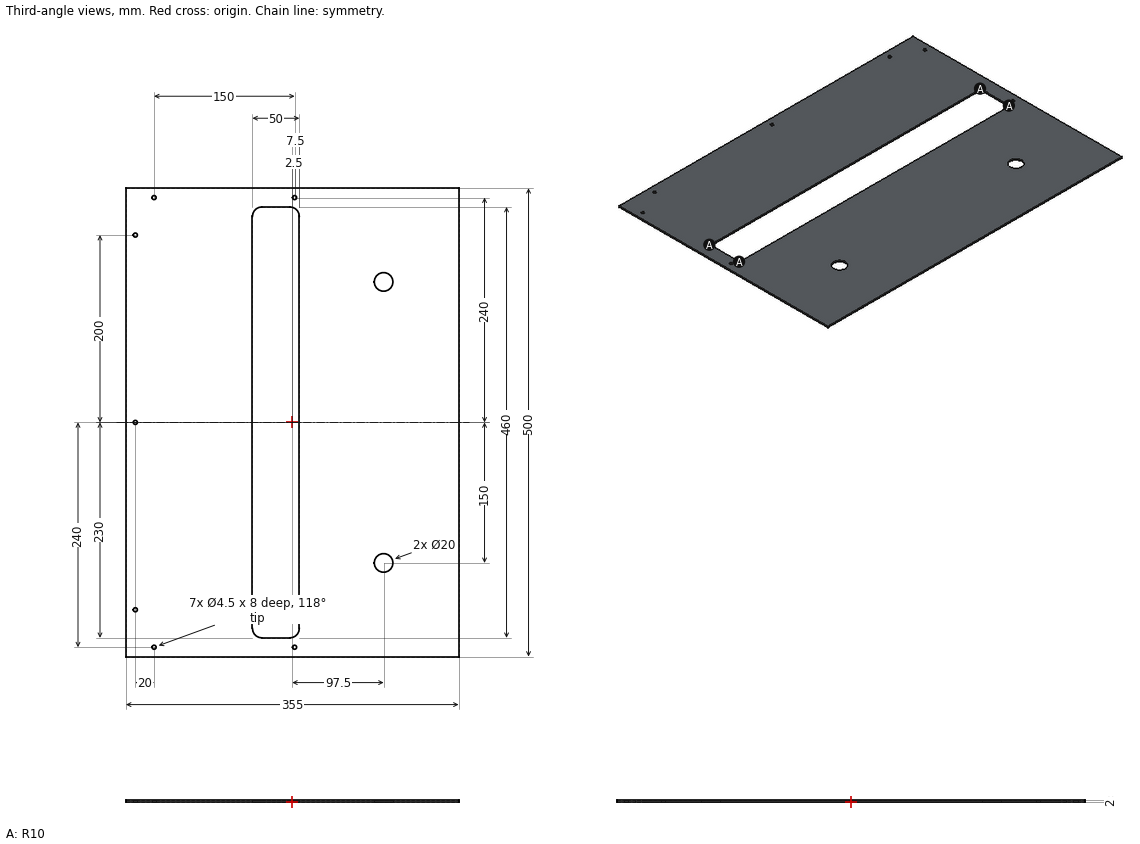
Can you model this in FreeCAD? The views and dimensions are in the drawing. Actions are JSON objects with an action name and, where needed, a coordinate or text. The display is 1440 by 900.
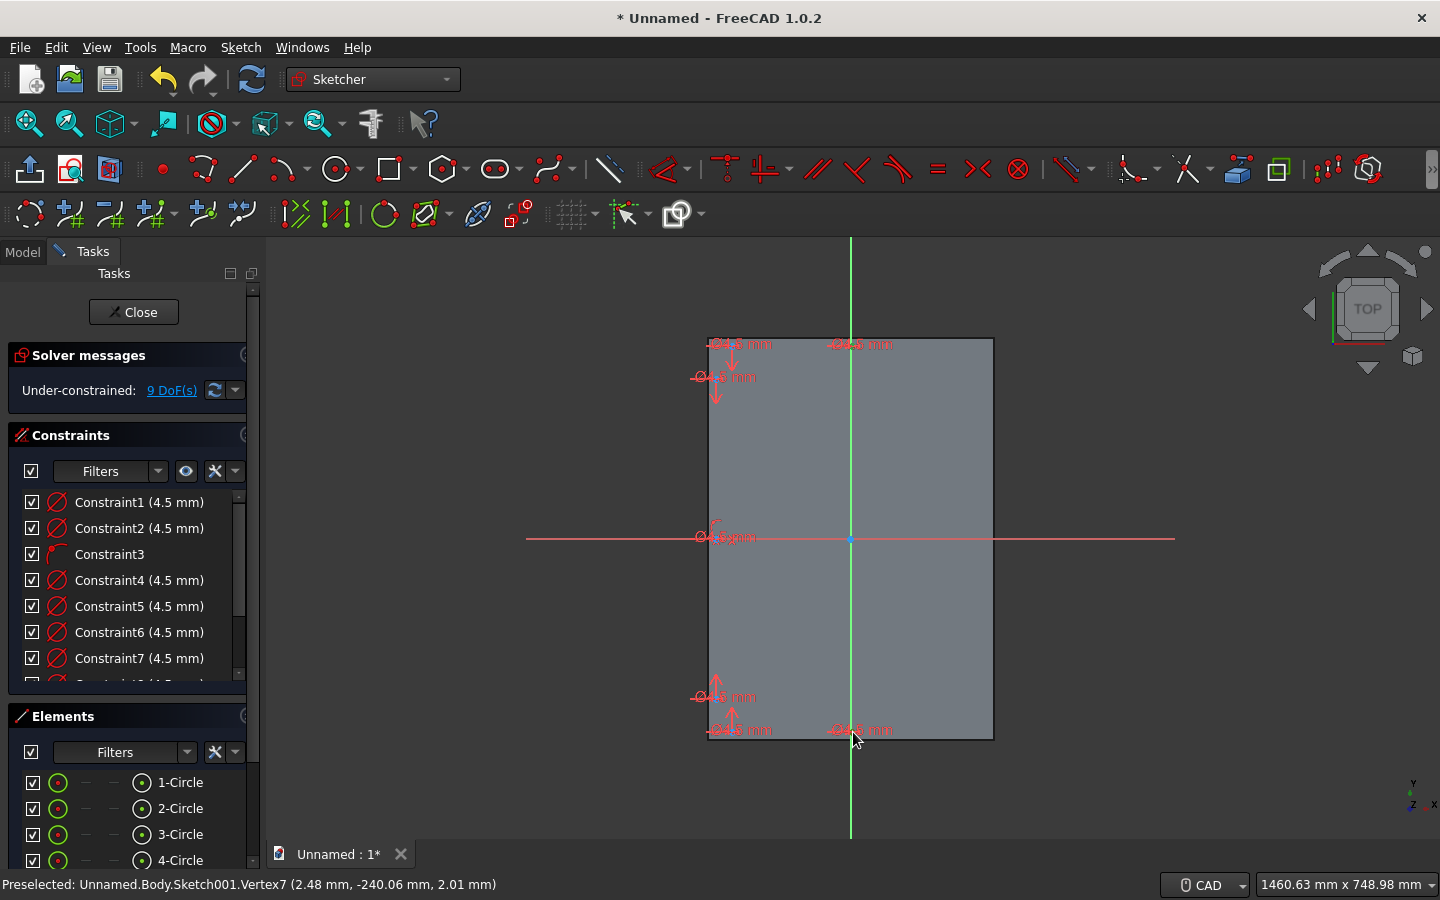
{"action": "left_click", "coordinate": [574, 539]}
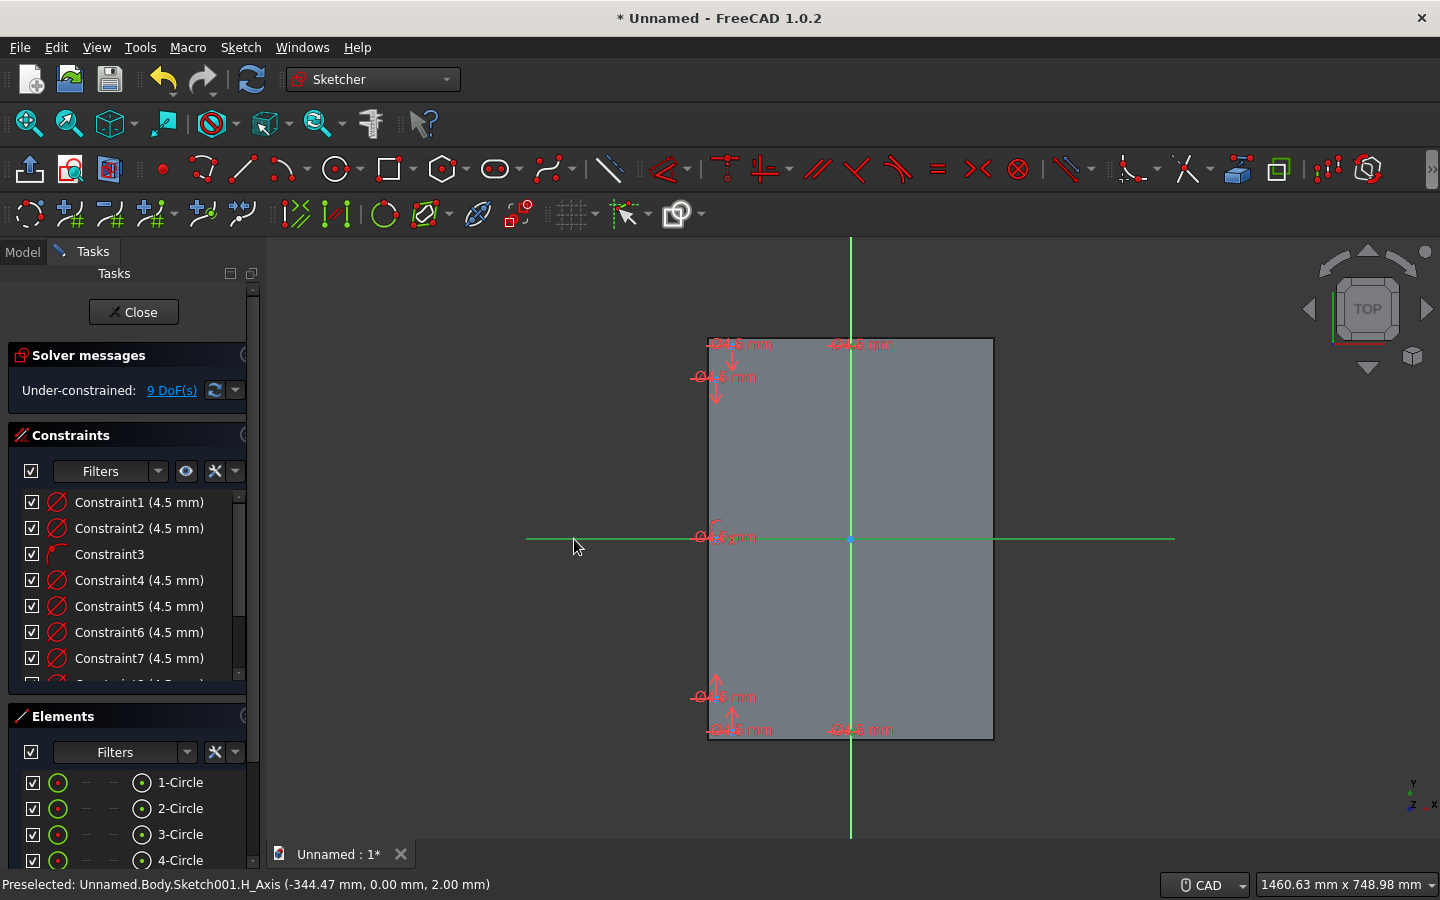
{"action": "key", "text": "s"}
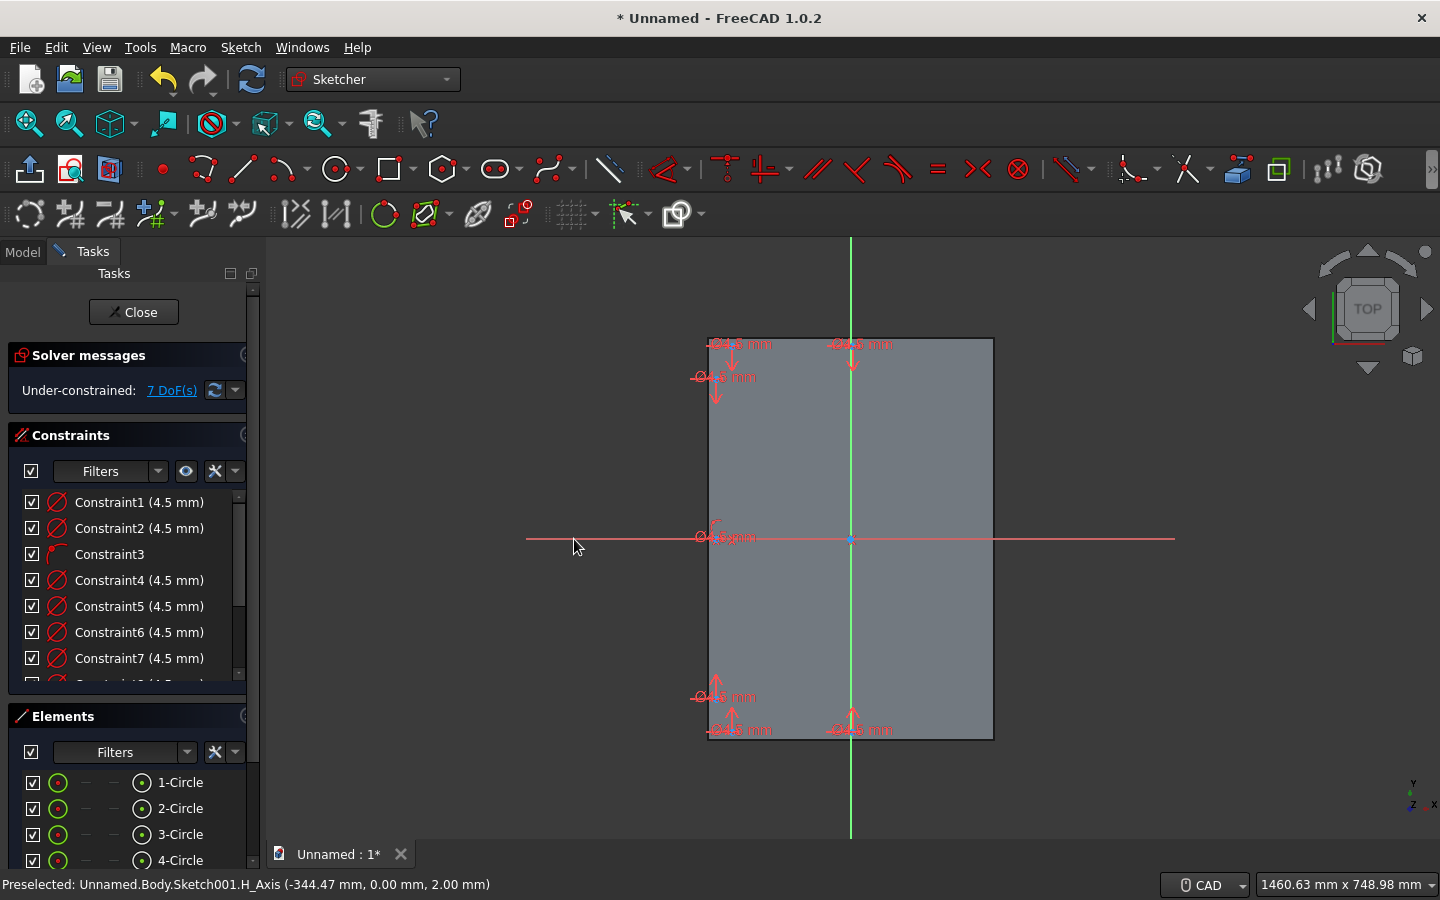
{"action": "left_click", "coordinate": [664, 170]}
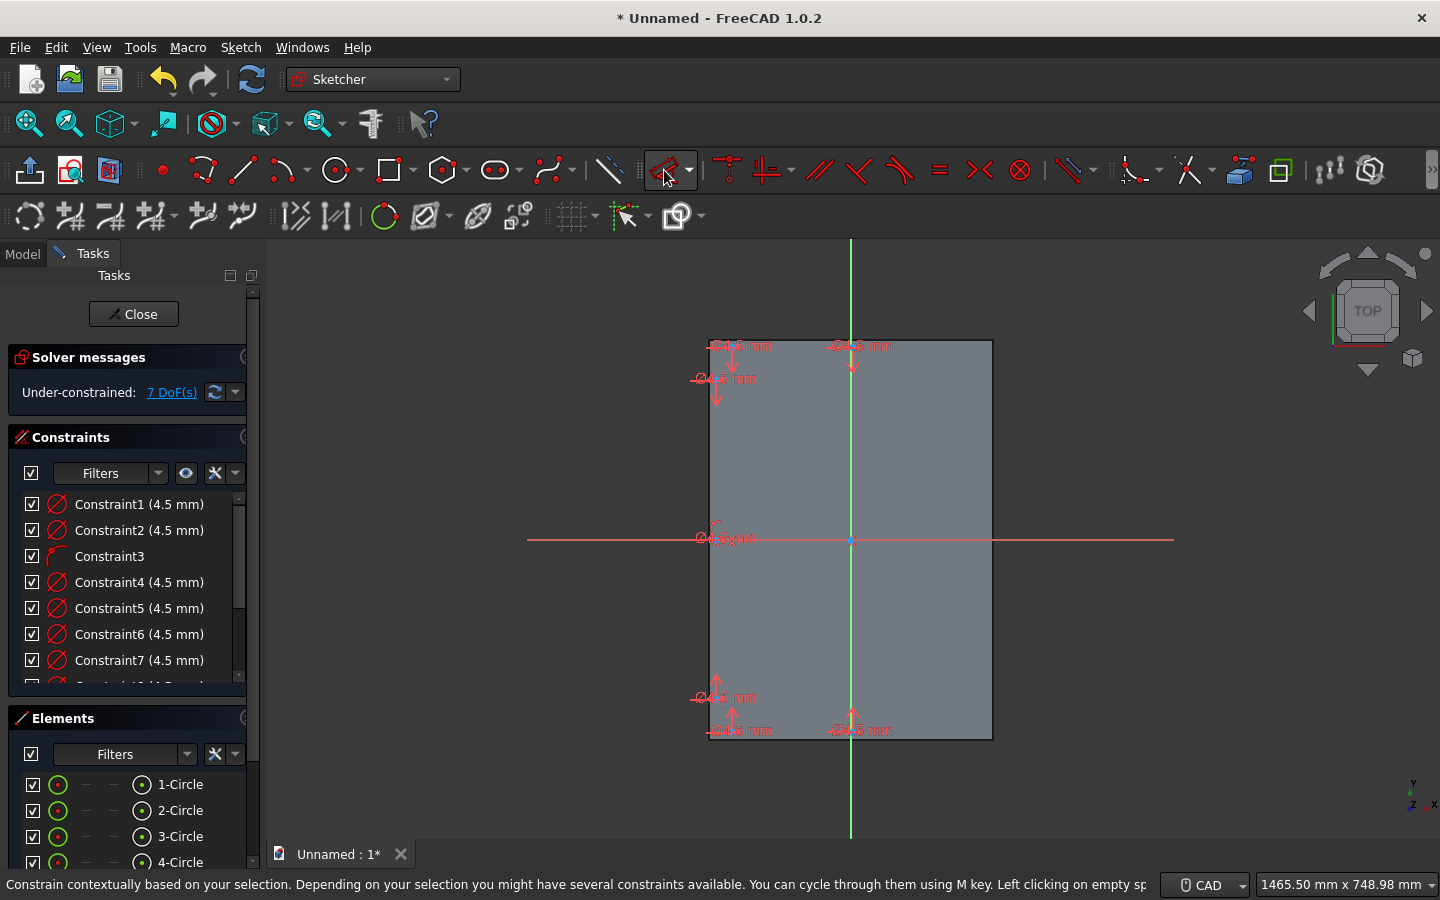
{"action": "left_click", "coordinate": [732, 733]}
{"action": "left_click", "coordinate": [885, 636]}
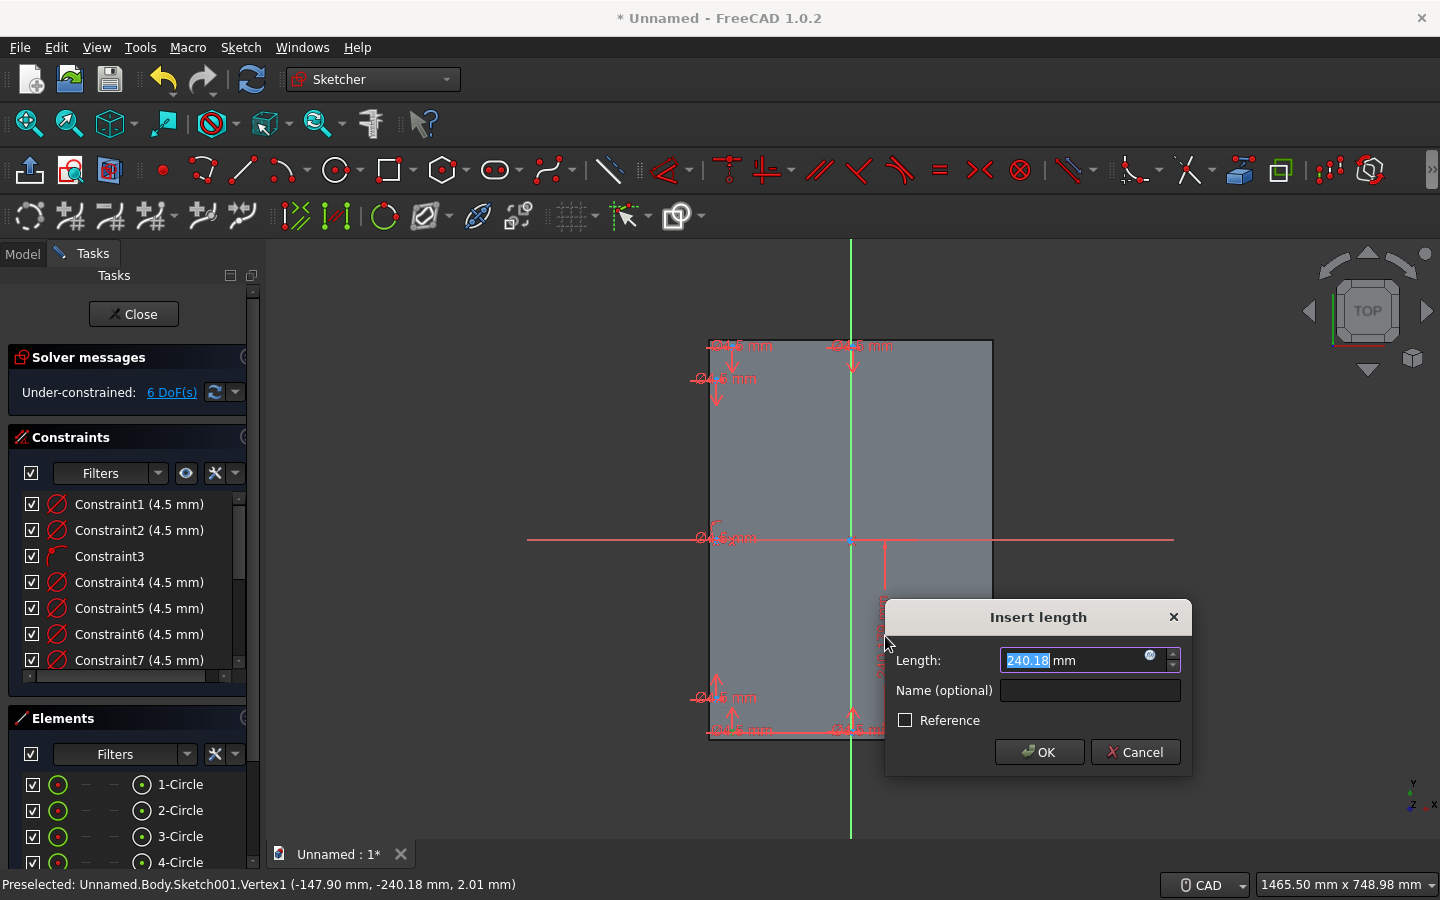
{"action": "type", "text": "240"}
{"action": "key", "text": "Return"}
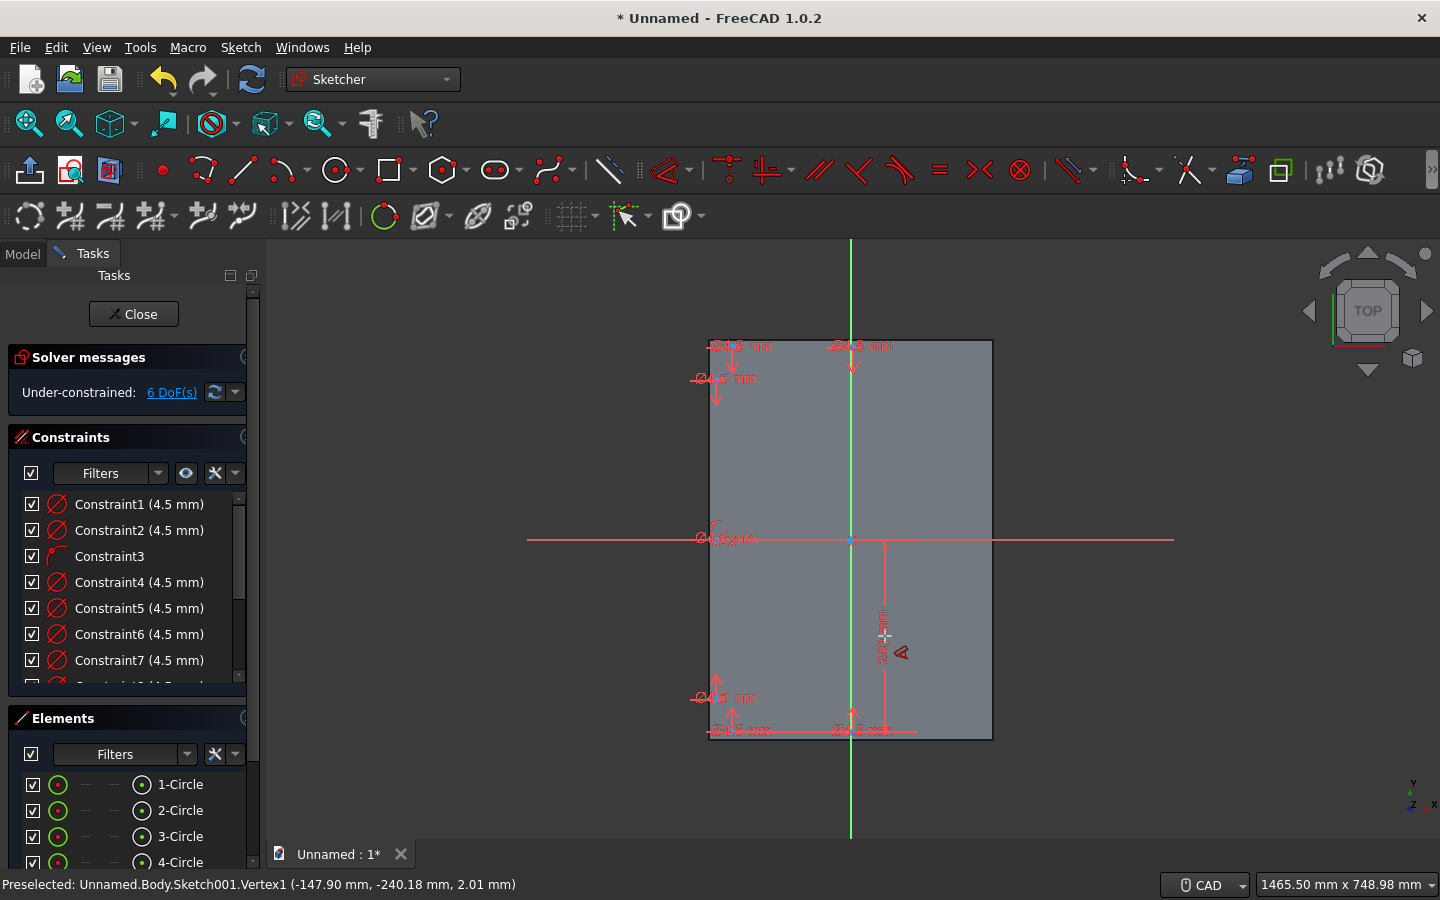
{"action": "left_click", "coordinate": [716, 381]}
{"action": "left_click", "coordinate": [682, 460]}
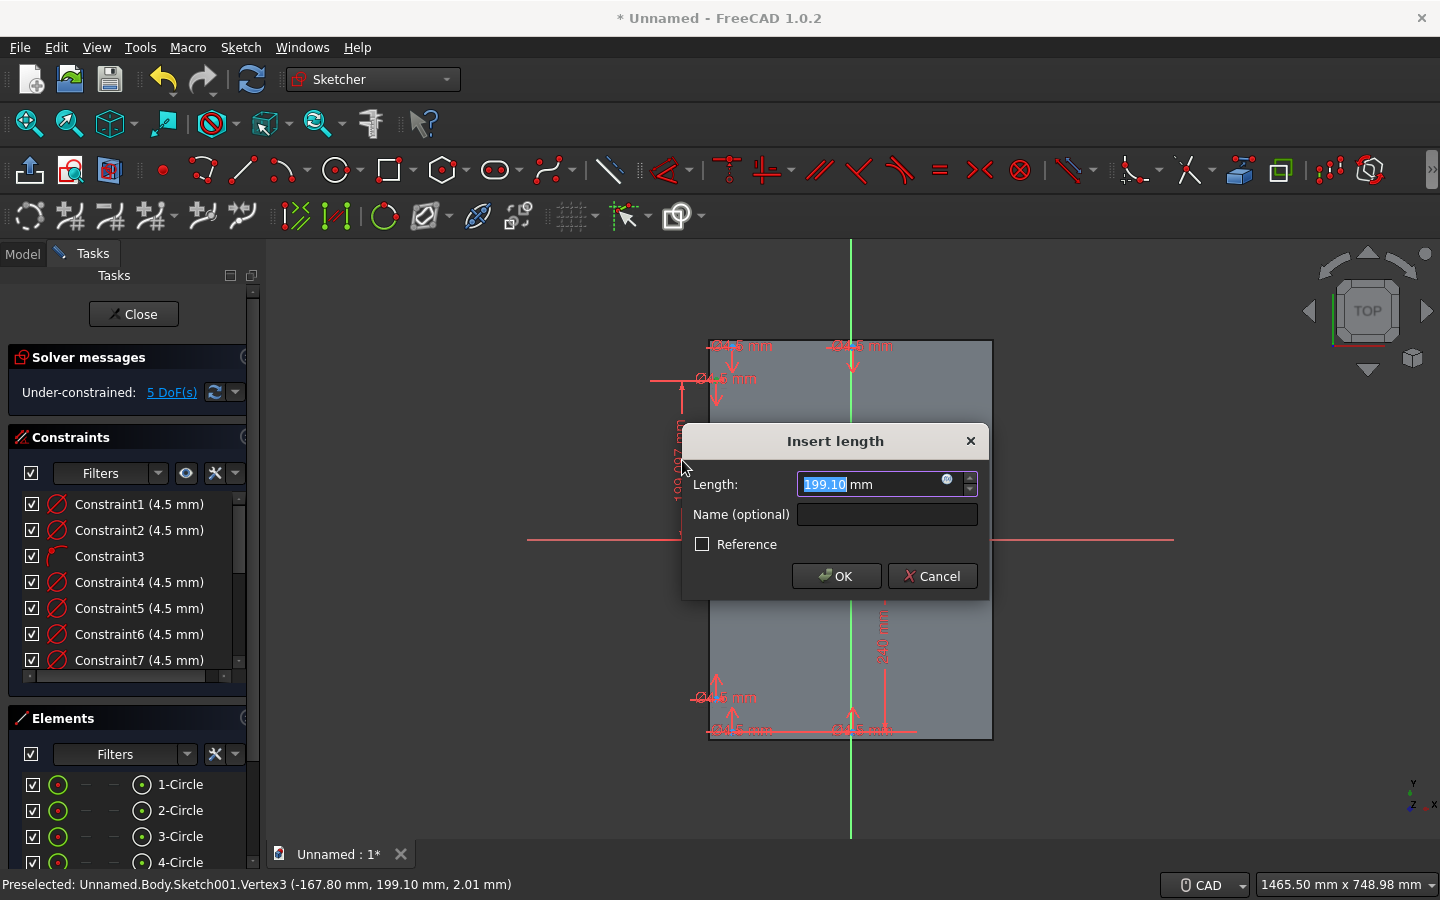
{"action": "type", "text": "200"}
{"action": "key", "text": "Return"}